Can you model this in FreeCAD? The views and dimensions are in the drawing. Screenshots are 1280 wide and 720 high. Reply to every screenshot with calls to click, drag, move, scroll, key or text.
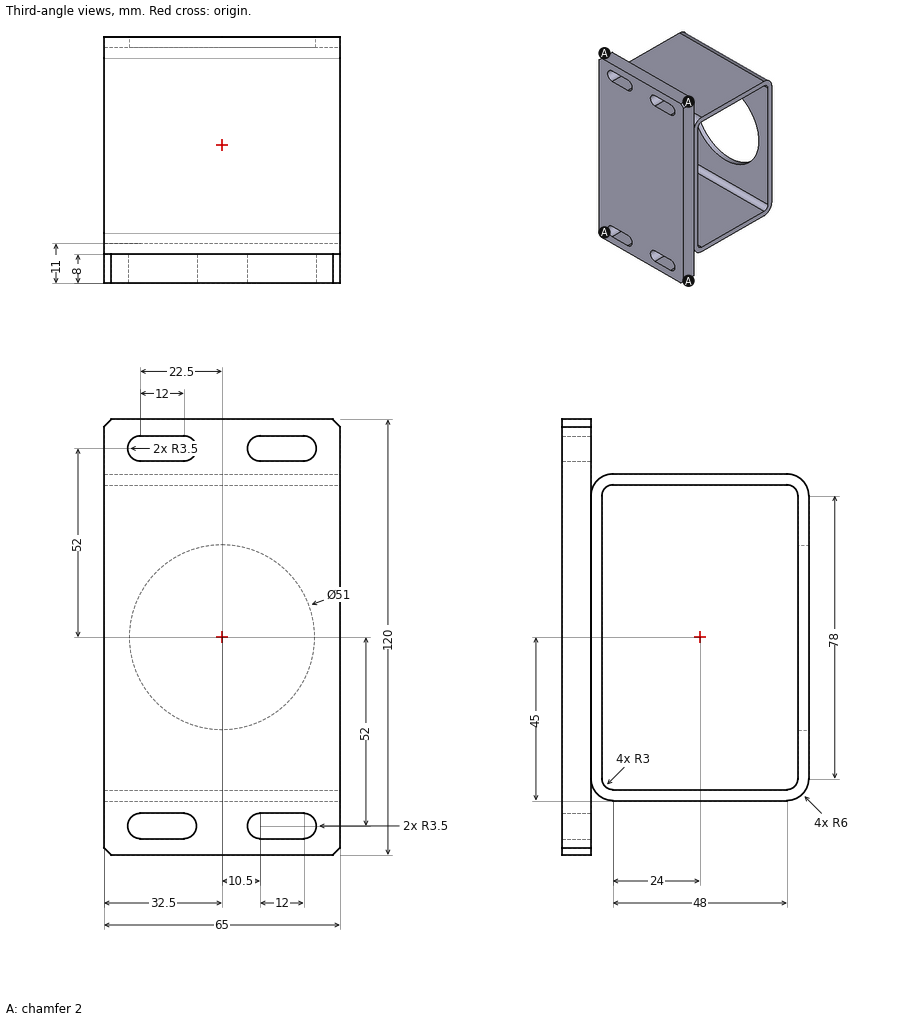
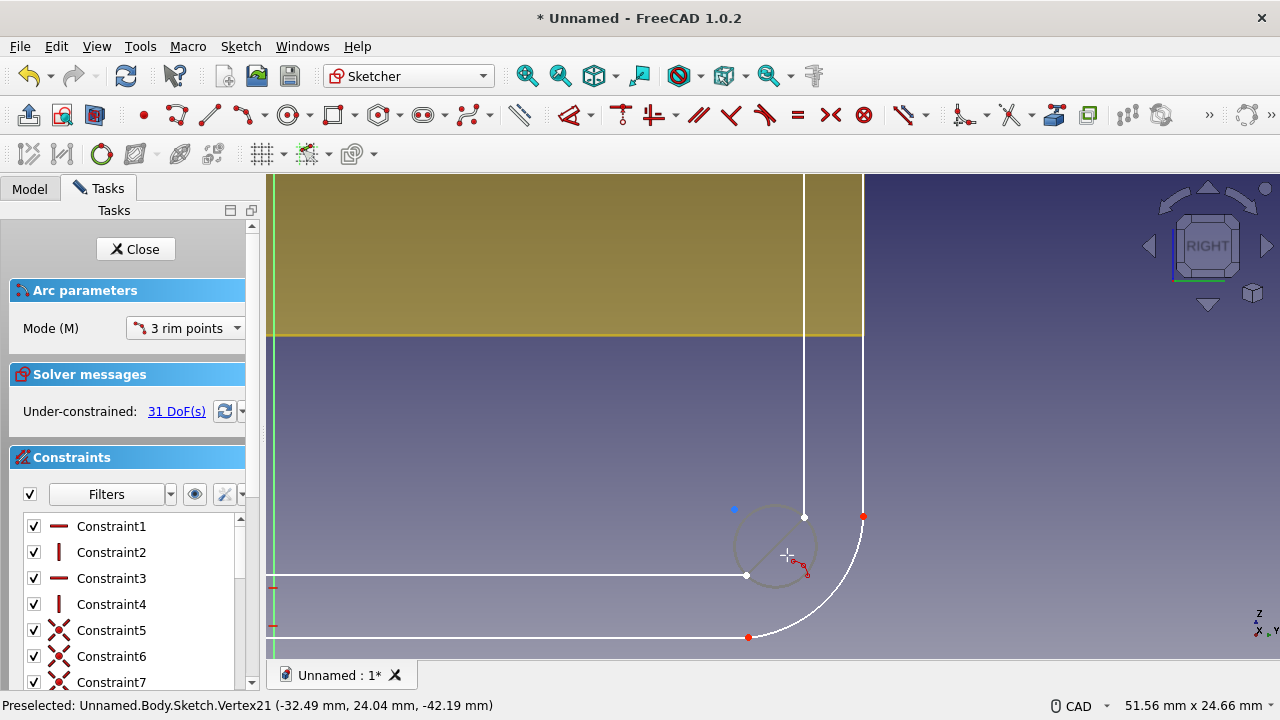
click(787, 554)
key(Escape)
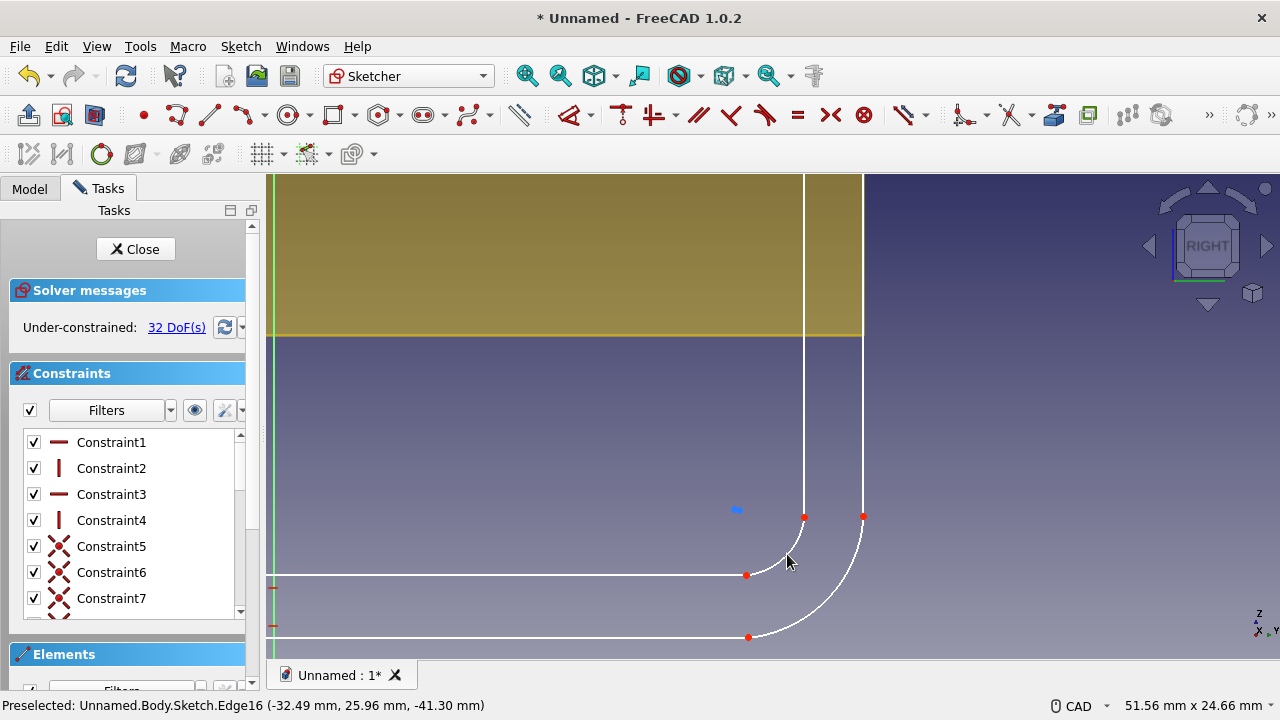
scroll(790, 549, down, 9)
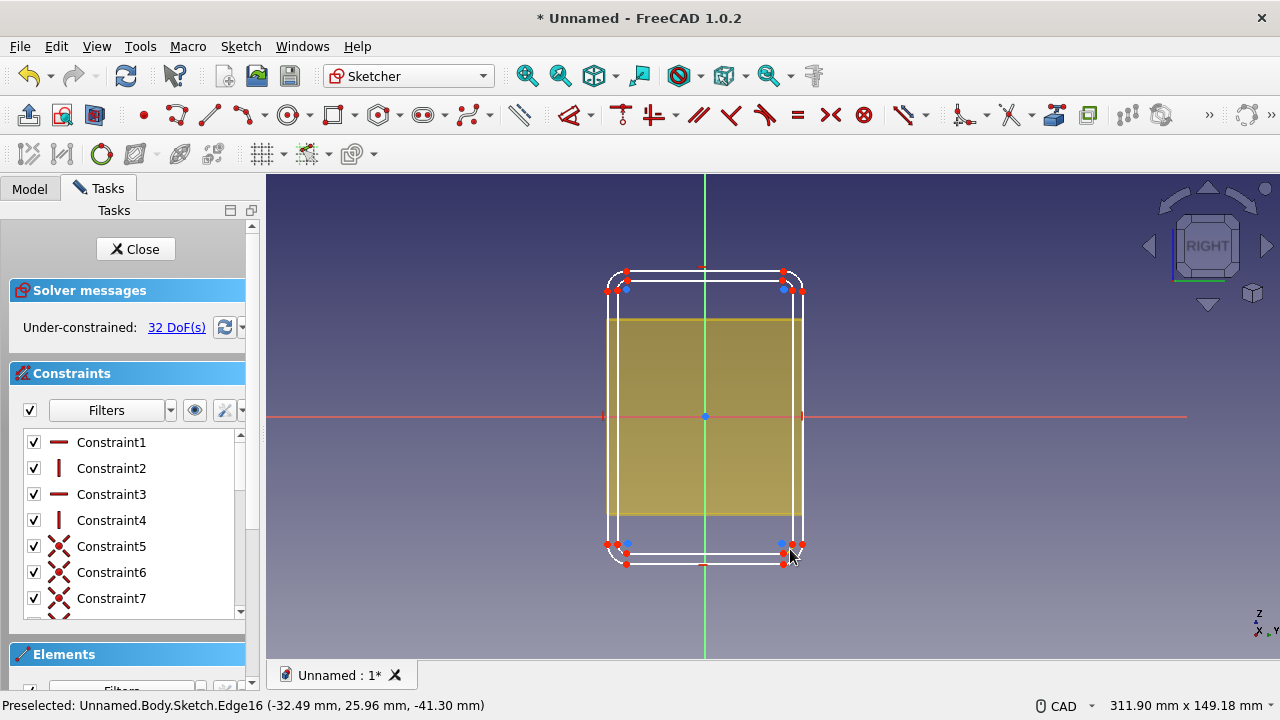
scroll(674, 564, up, 2)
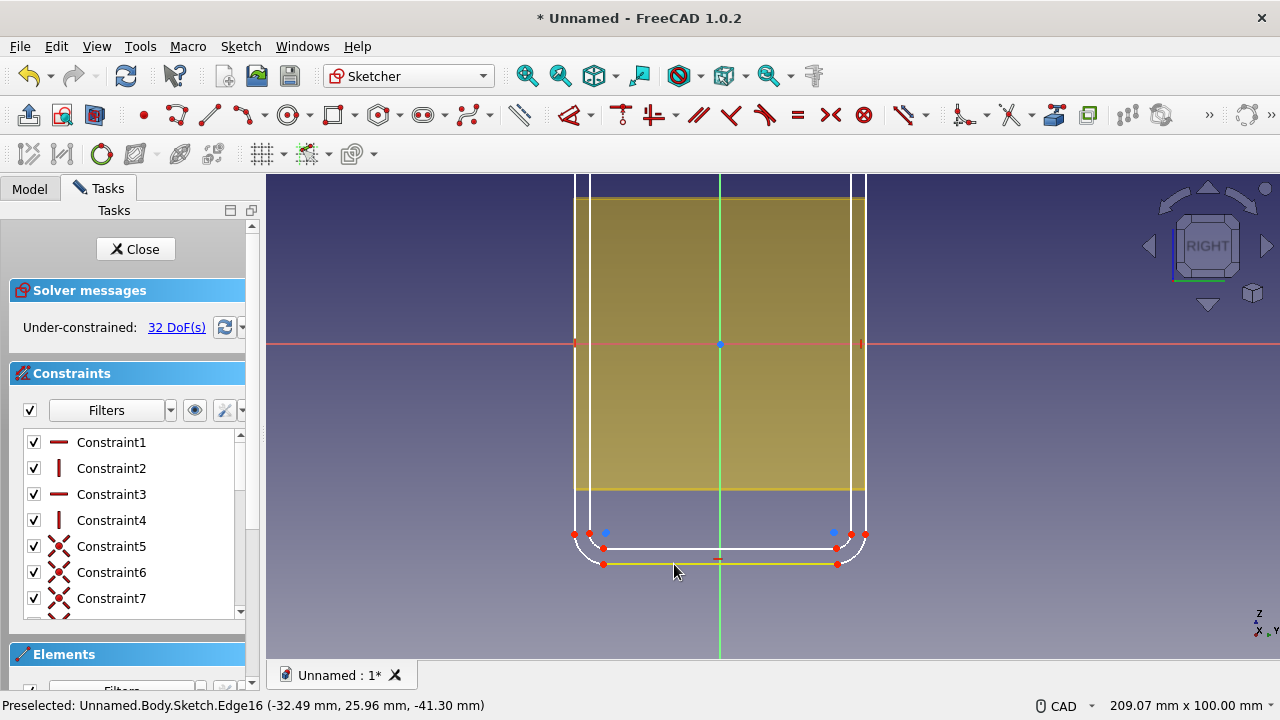
click(673, 564)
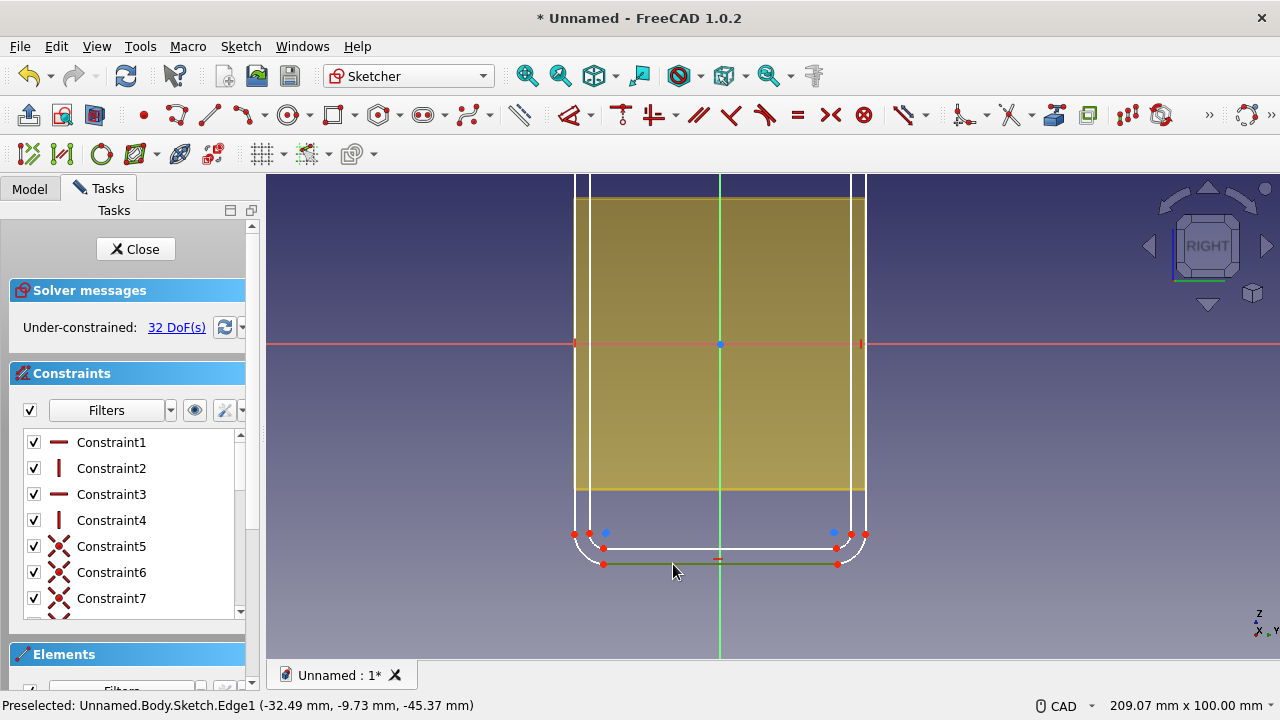
click(850, 560)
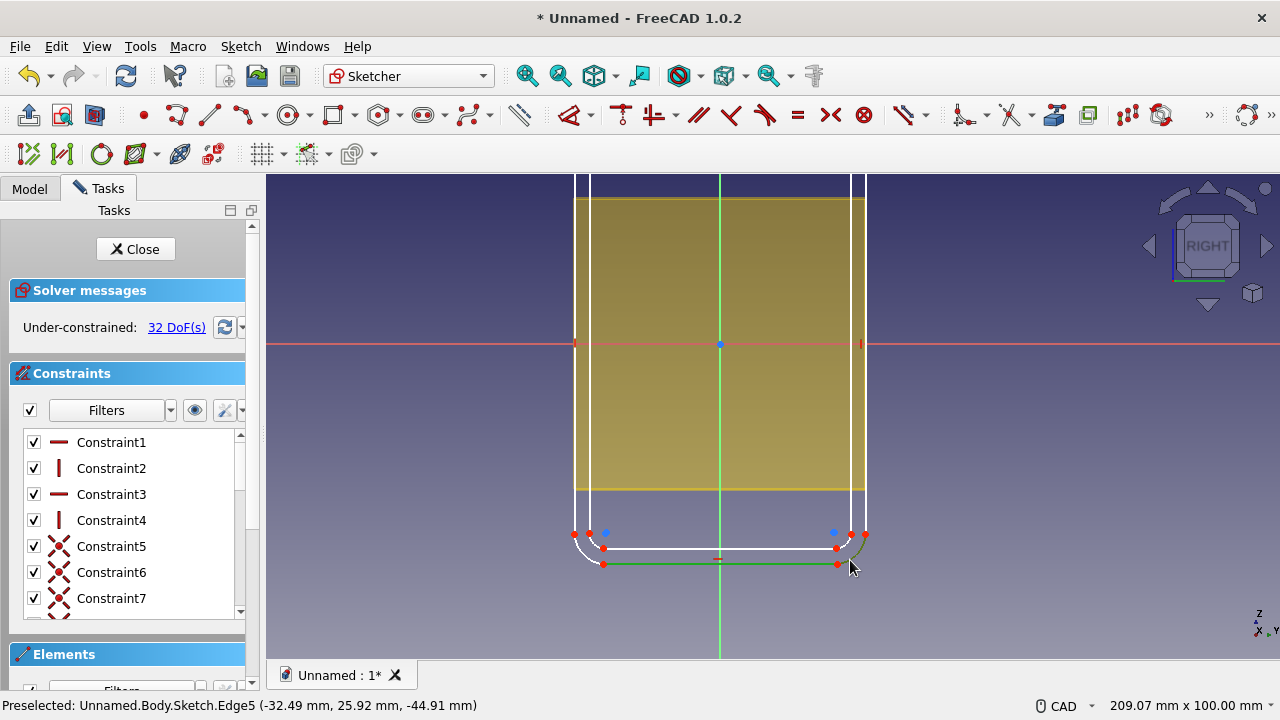
click(765, 116)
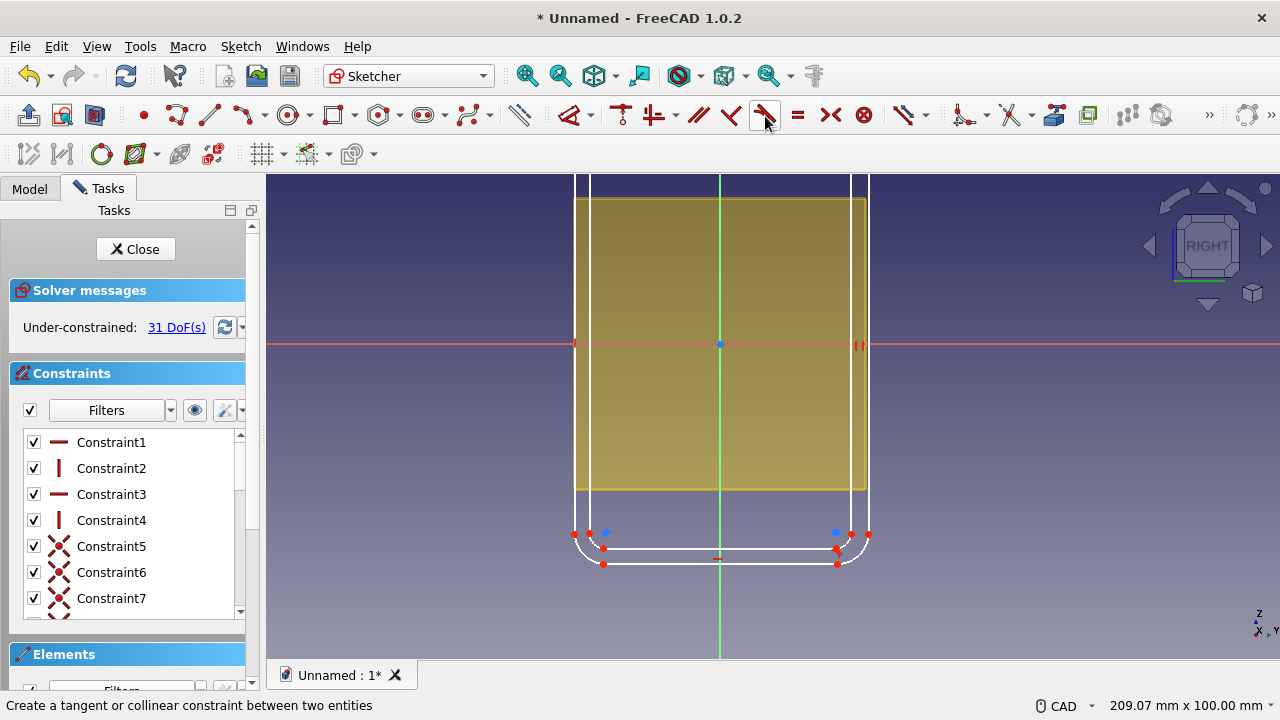
click(673, 564)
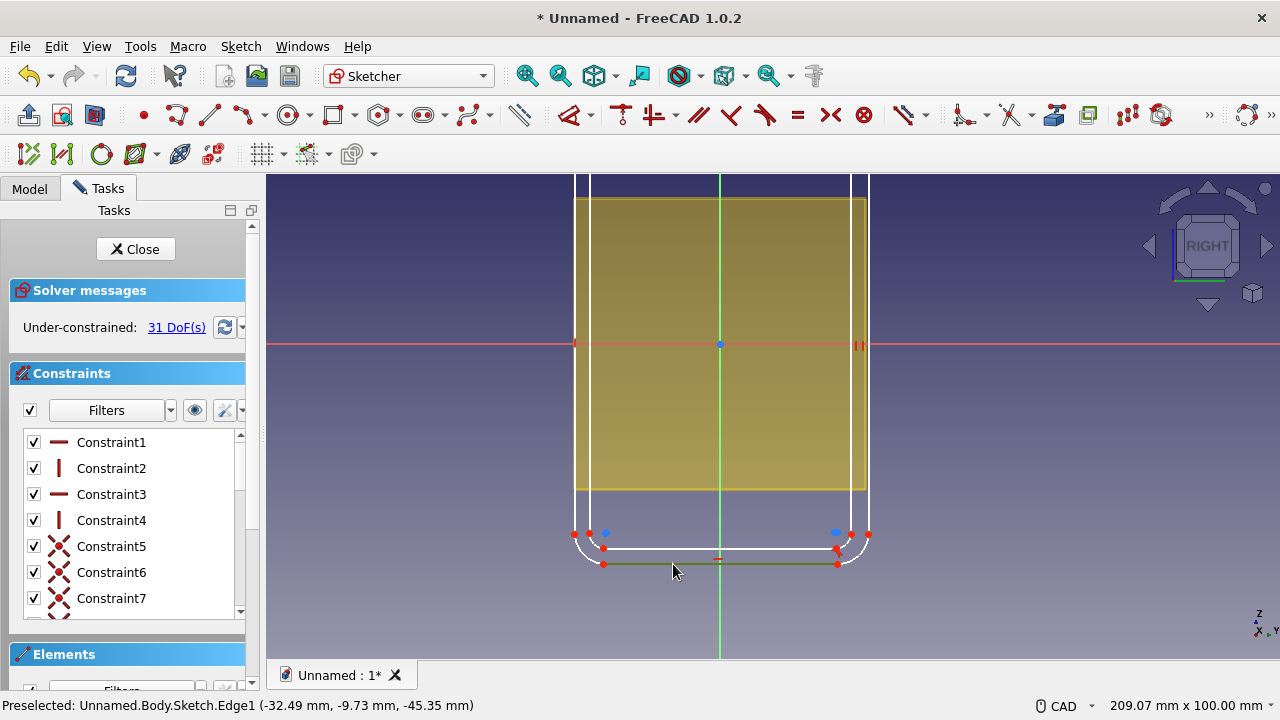
click(578, 547)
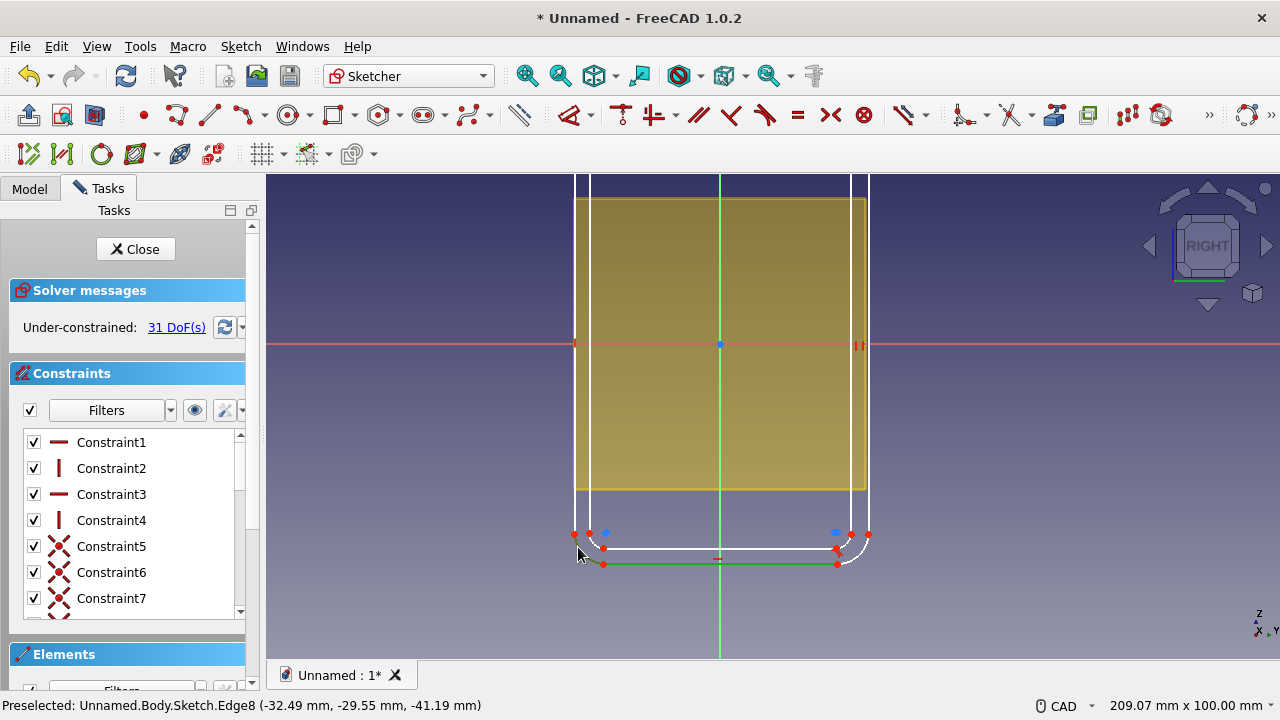
click(765, 116)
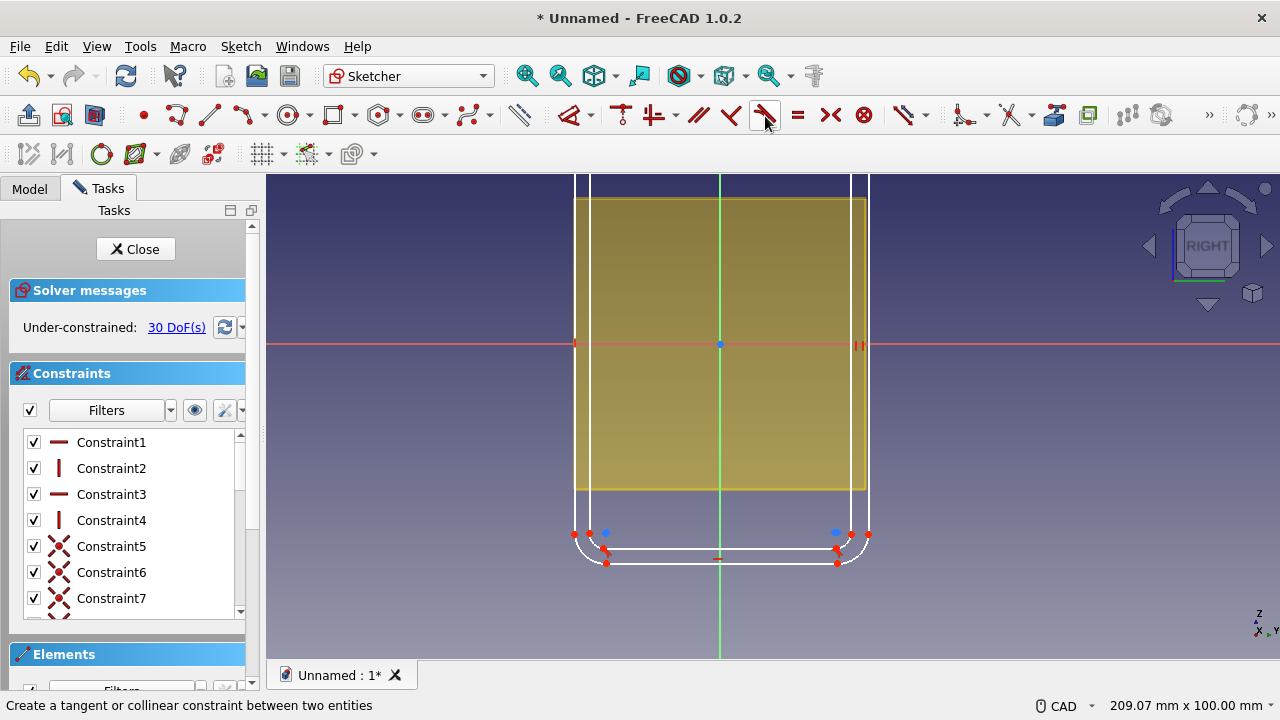
click(869, 421)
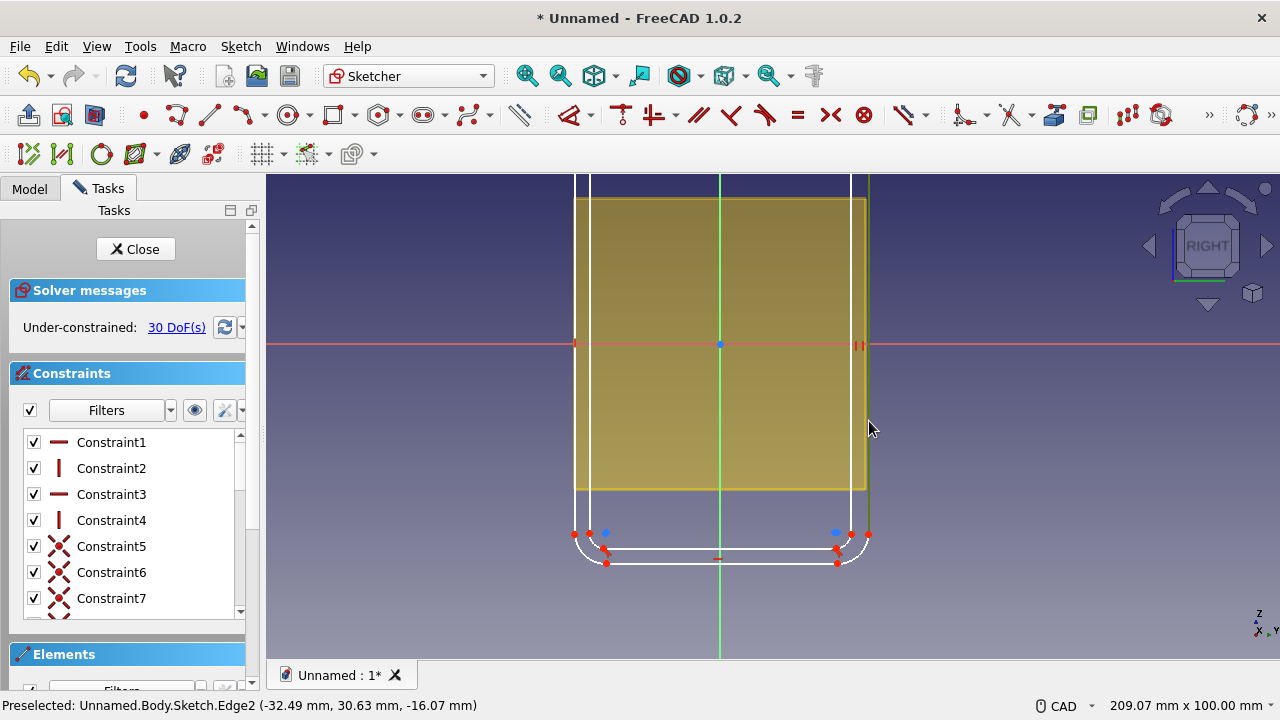
click(851, 561)